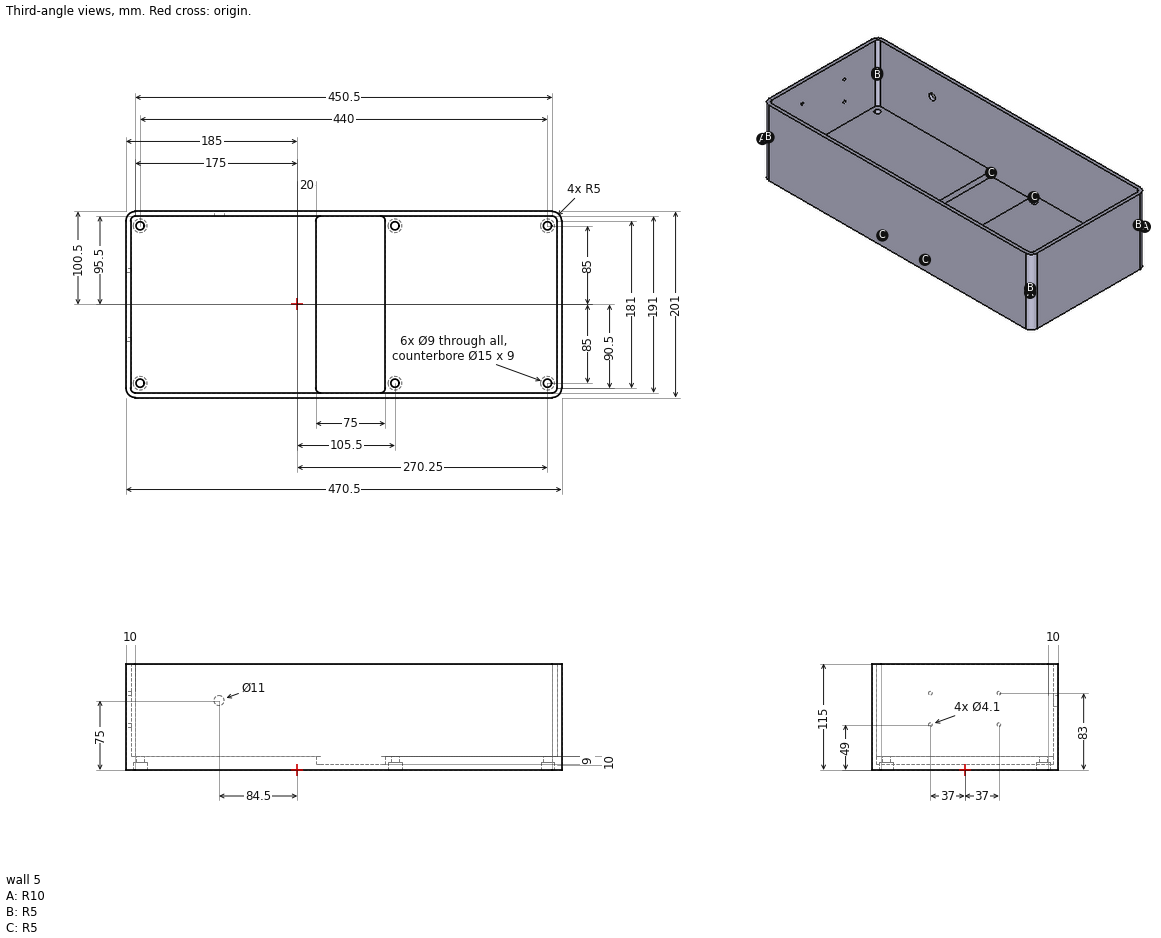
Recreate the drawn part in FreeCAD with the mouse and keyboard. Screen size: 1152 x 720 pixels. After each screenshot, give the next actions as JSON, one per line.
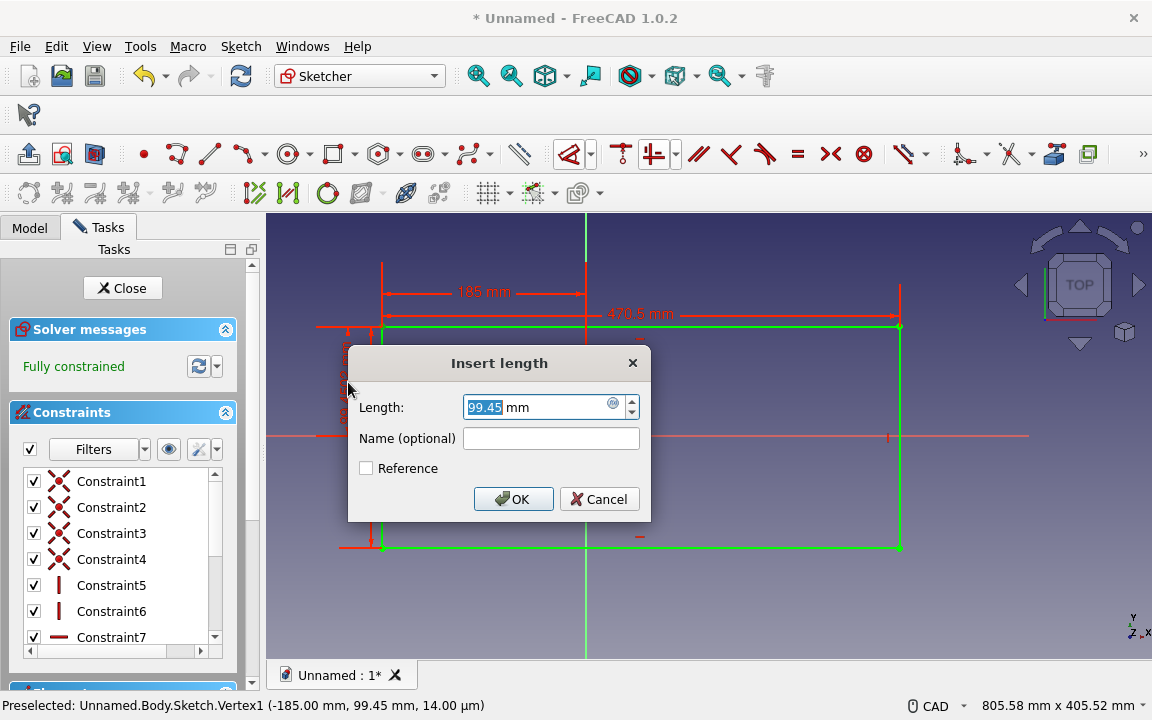
{"action": "type", "text": "100.5"}
{"action": "key", "text": "Return"}
{"action": "key", "text": "Escape"}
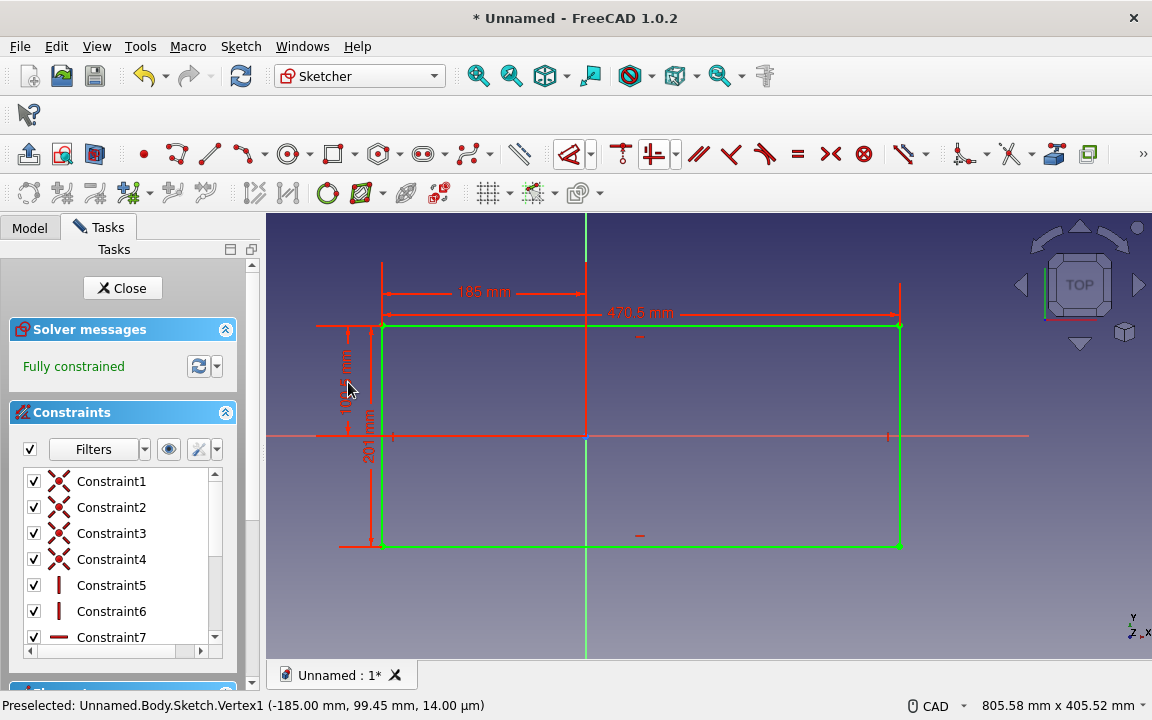
{"action": "left_click", "coordinate": [123, 288]}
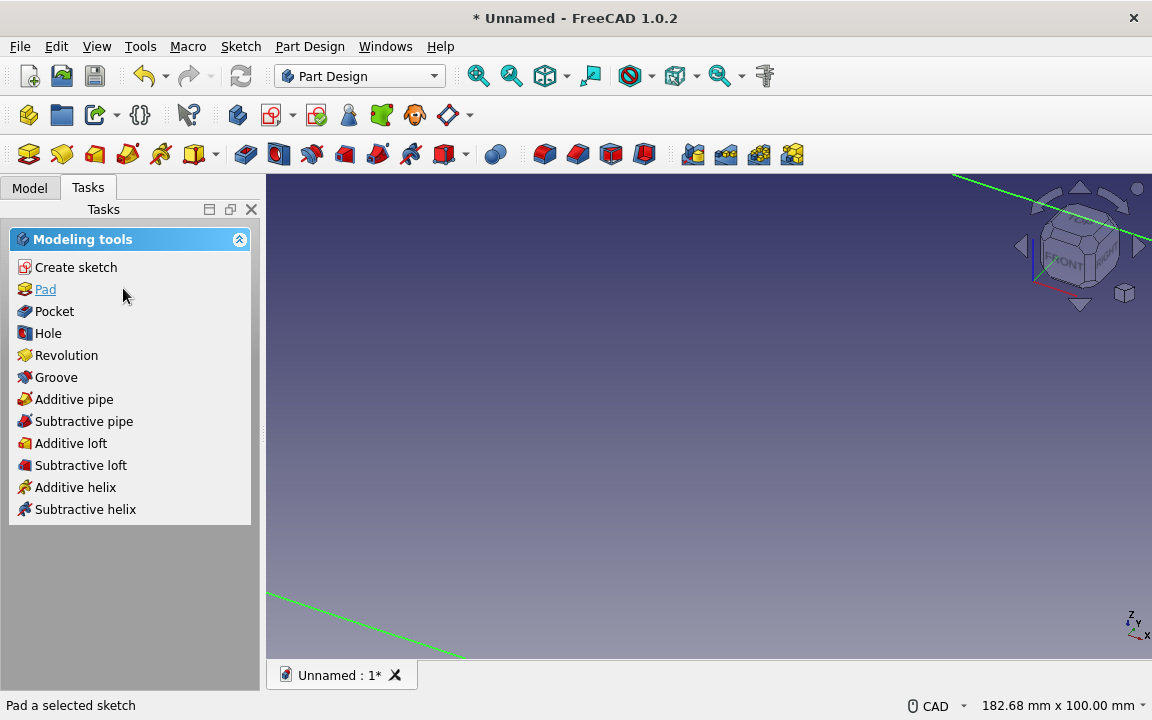
{"action": "left_click", "coordinate": [29, 154]}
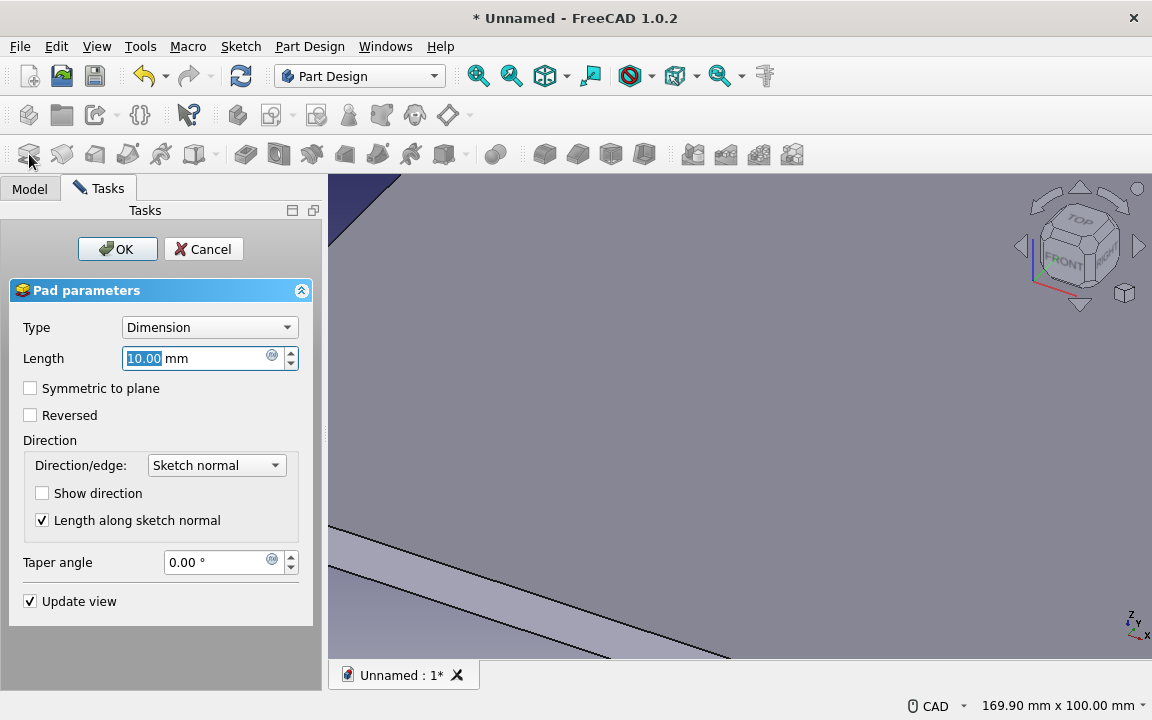
{"action": "type", "text": "115"}
{"action": "key", "text": "Tab"}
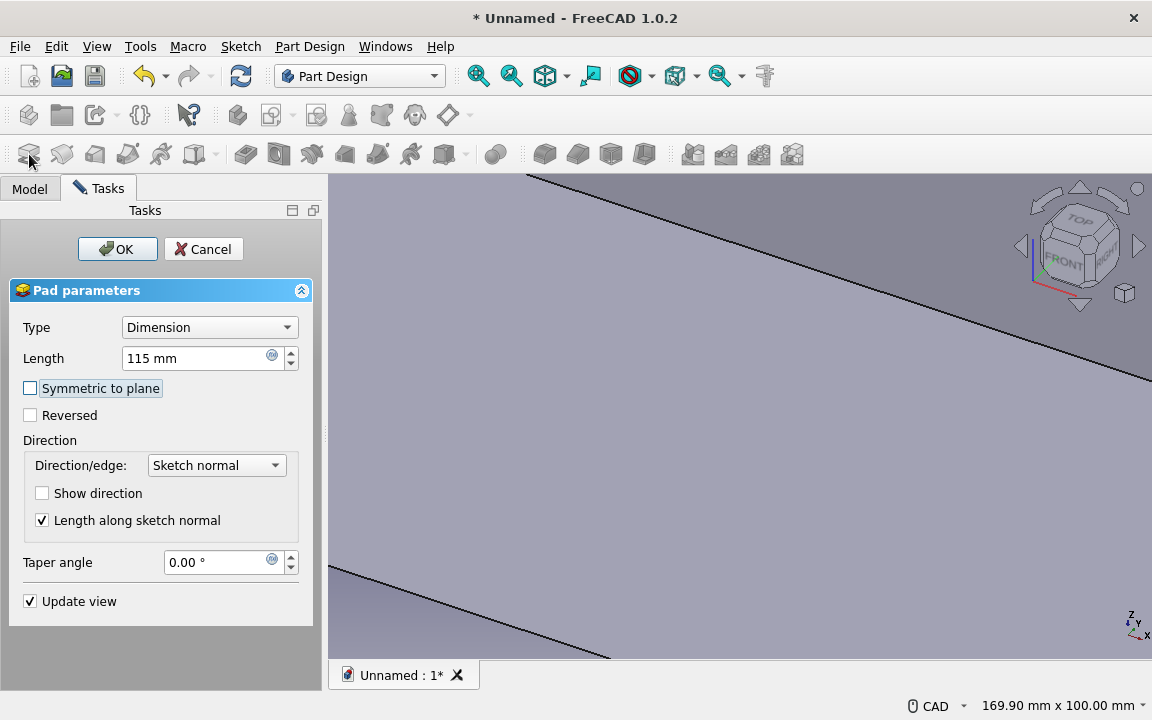
{"action": "left_click", "coordinate": [118, 249]}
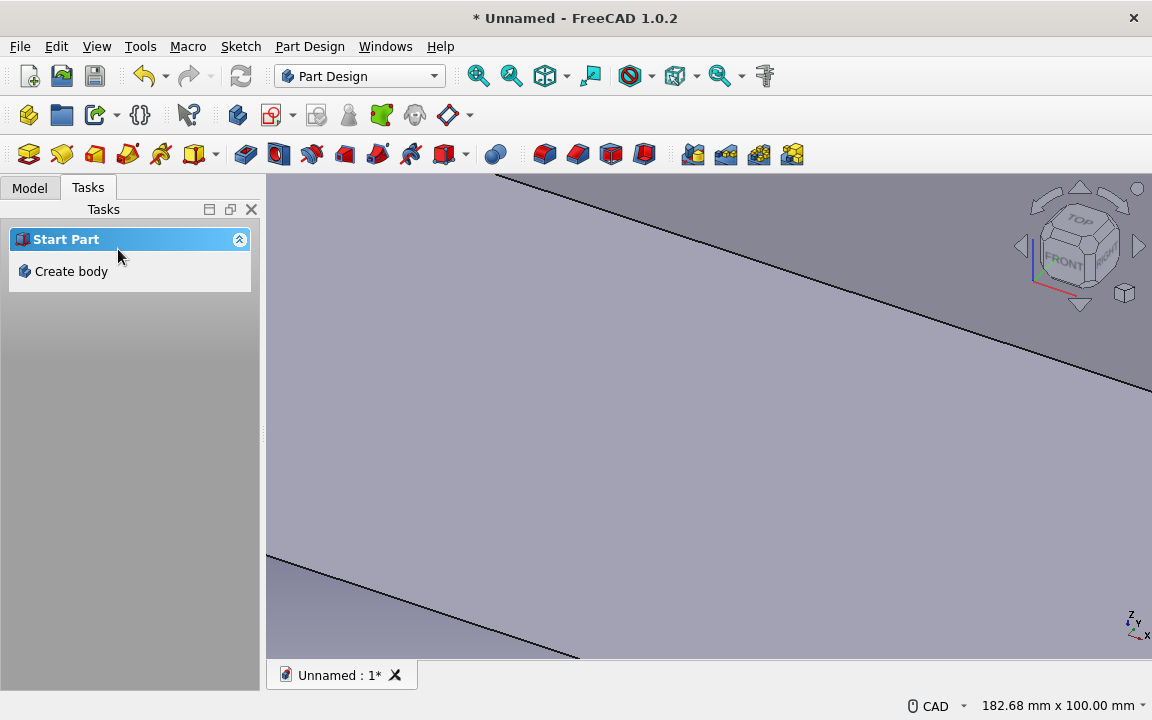
{"action": "key", "text": "v f"}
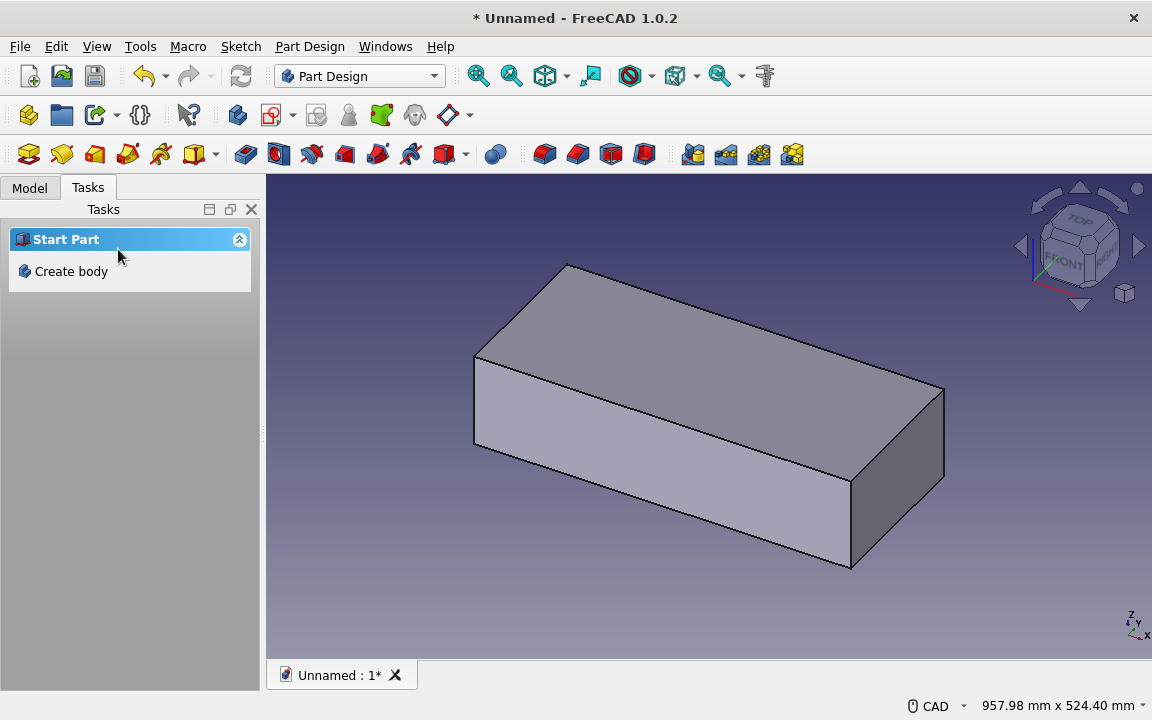
{"action": "left_click", "coordinate": [817, 408]}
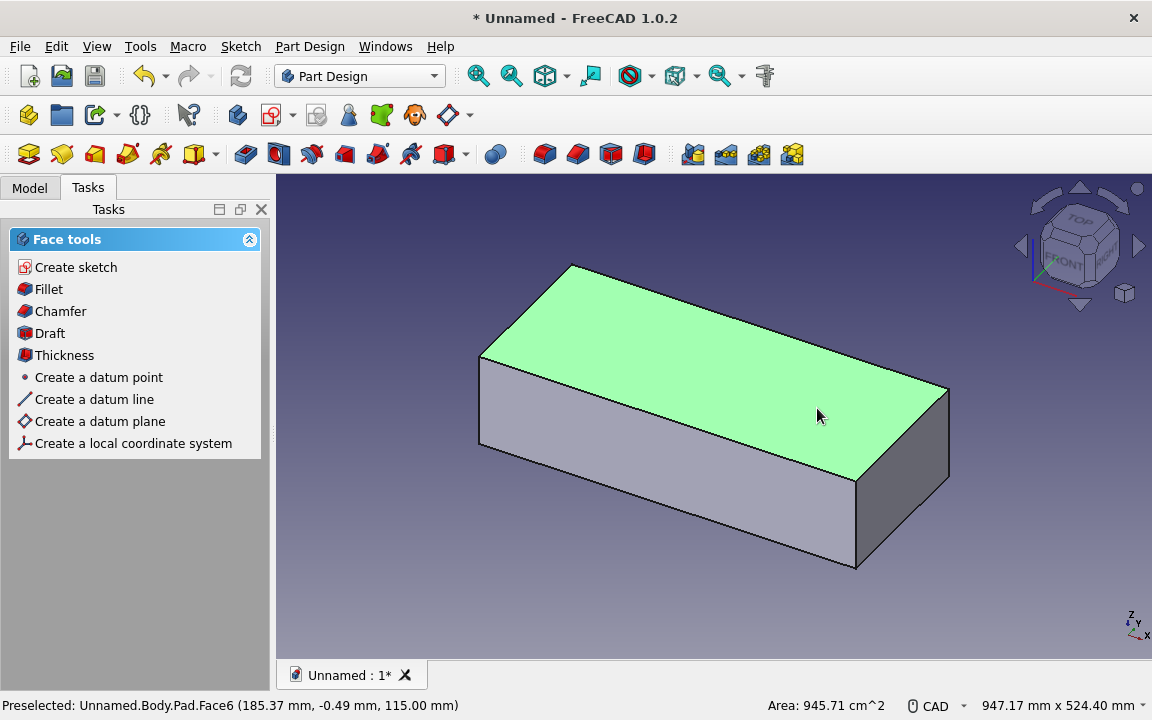
{"action": "left_click", "coordinate": [644, 154]}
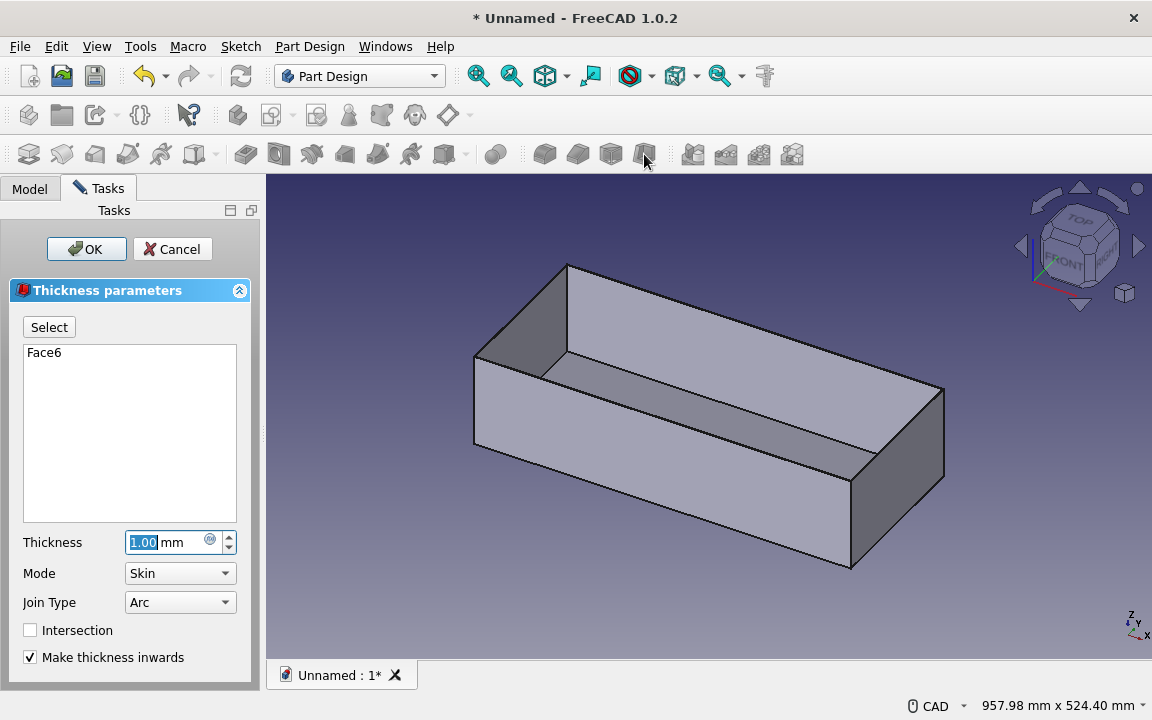
{"action": "type", "text": "5"}
{"action": "key", "text": "Tab"}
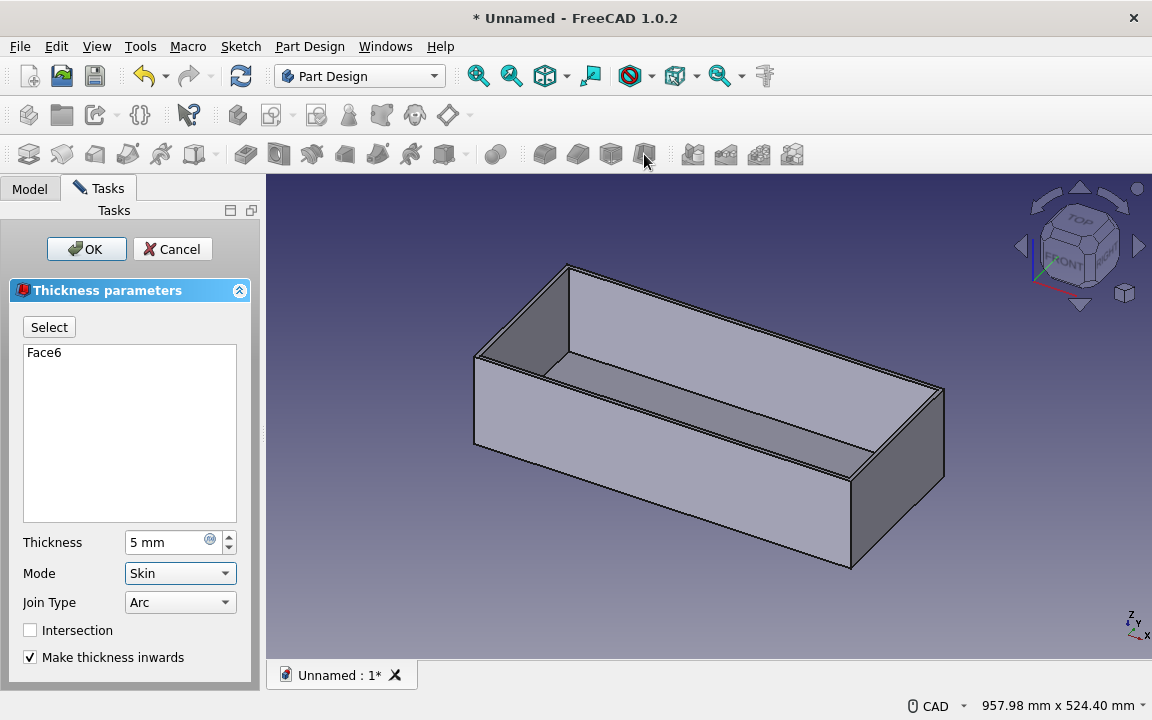
{"action": "left_click", "coordinate": [181, 602]}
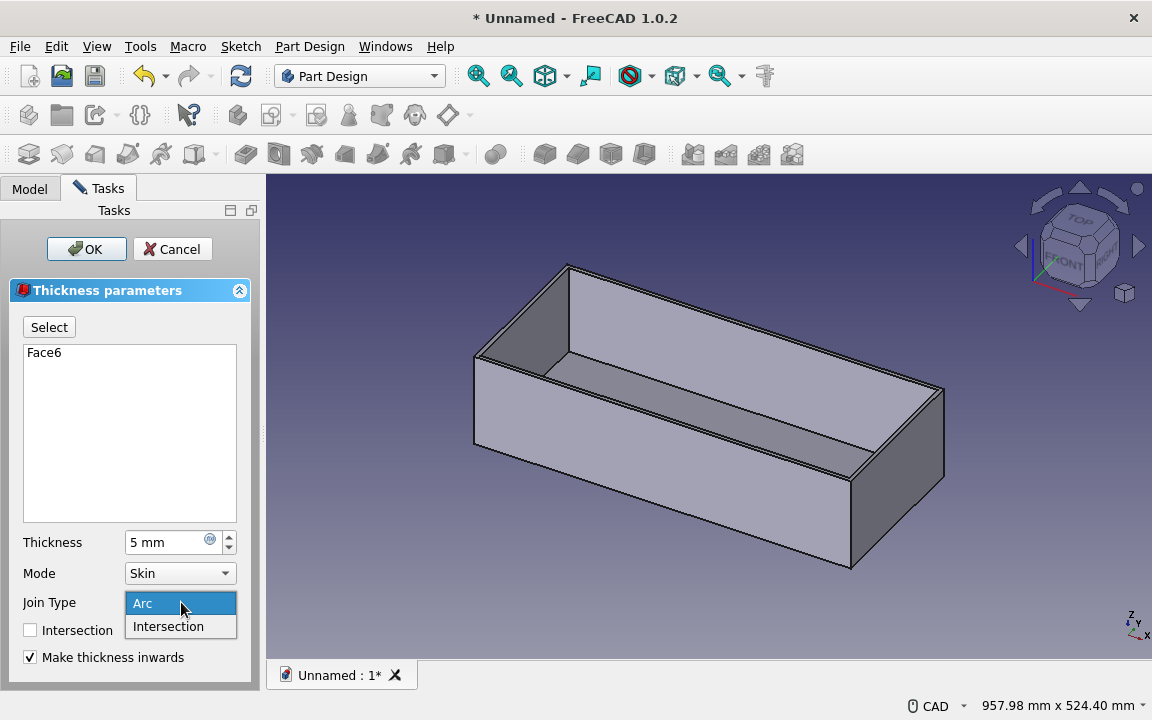
{"action": "left_click", "coordinate": [179, 626]}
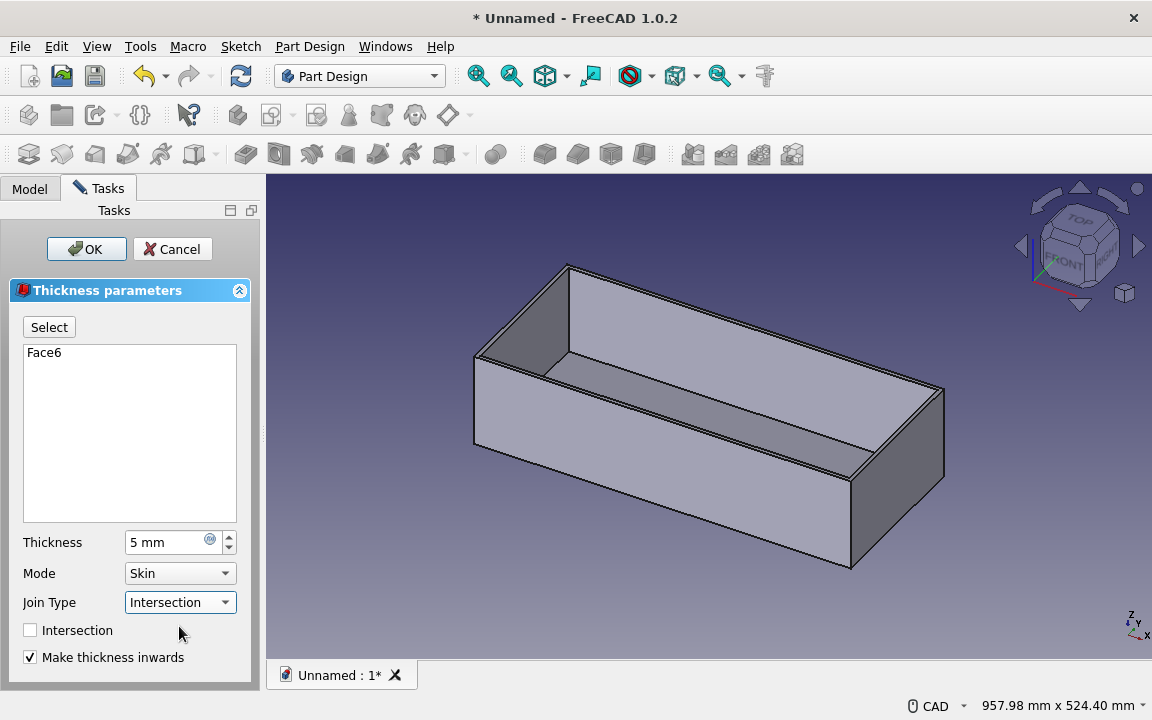
{"action": "left_click", "coordinate": [87, 249]}